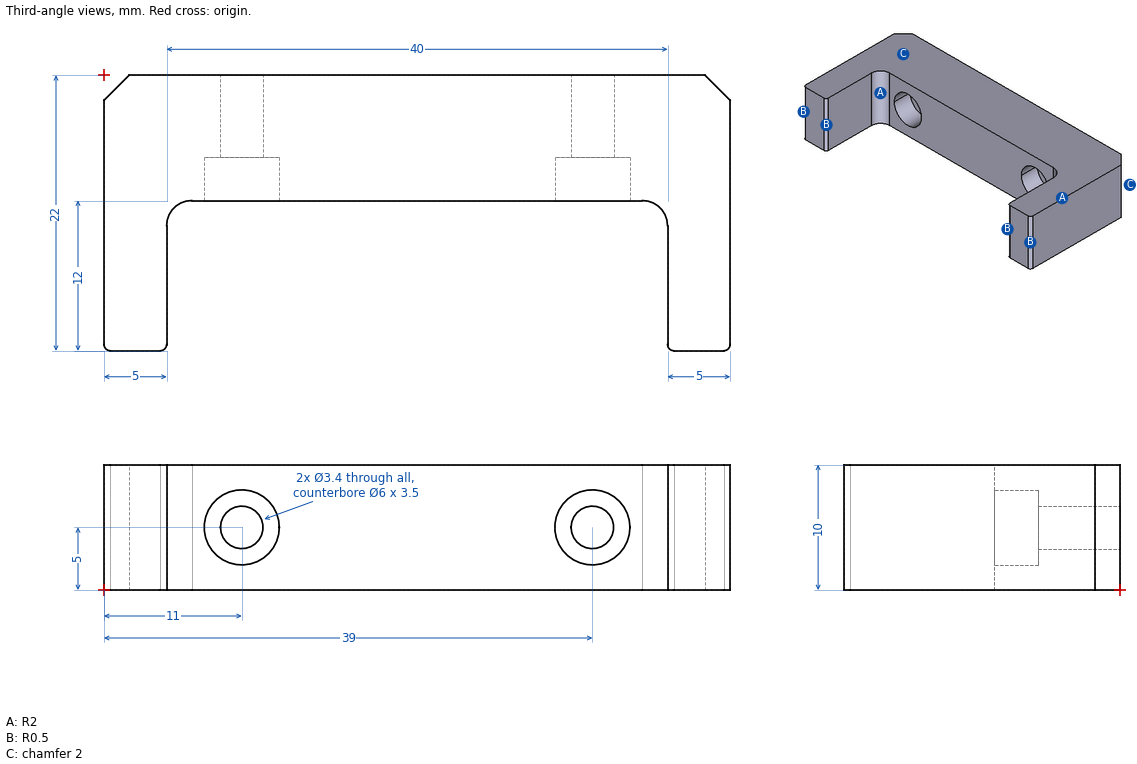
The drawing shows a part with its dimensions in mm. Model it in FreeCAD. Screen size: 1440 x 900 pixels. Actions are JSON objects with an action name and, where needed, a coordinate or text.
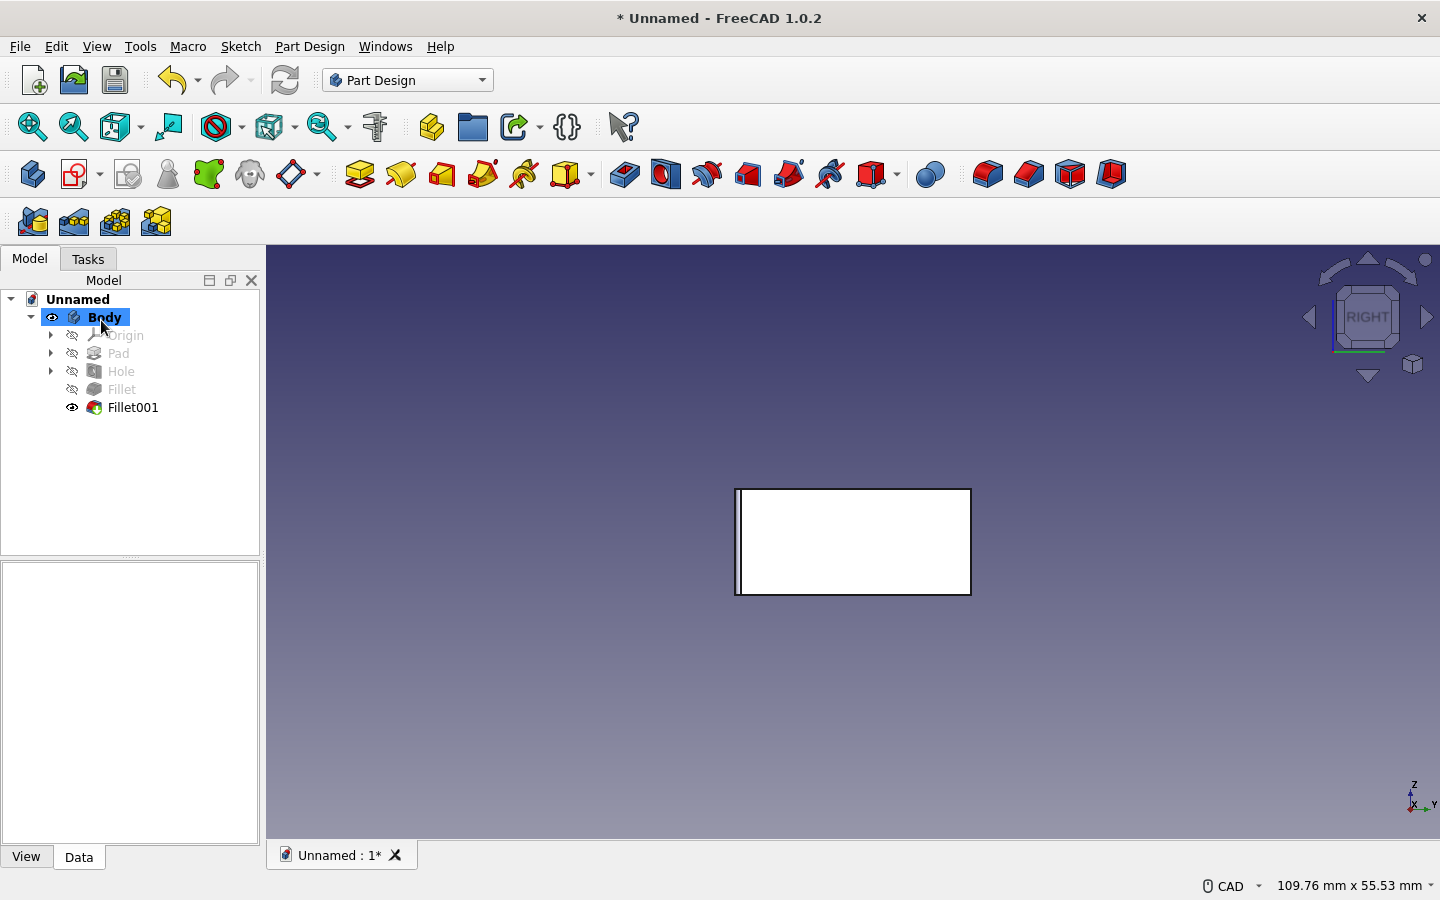
{"action": "left_click", "coordinate": [33, 128]}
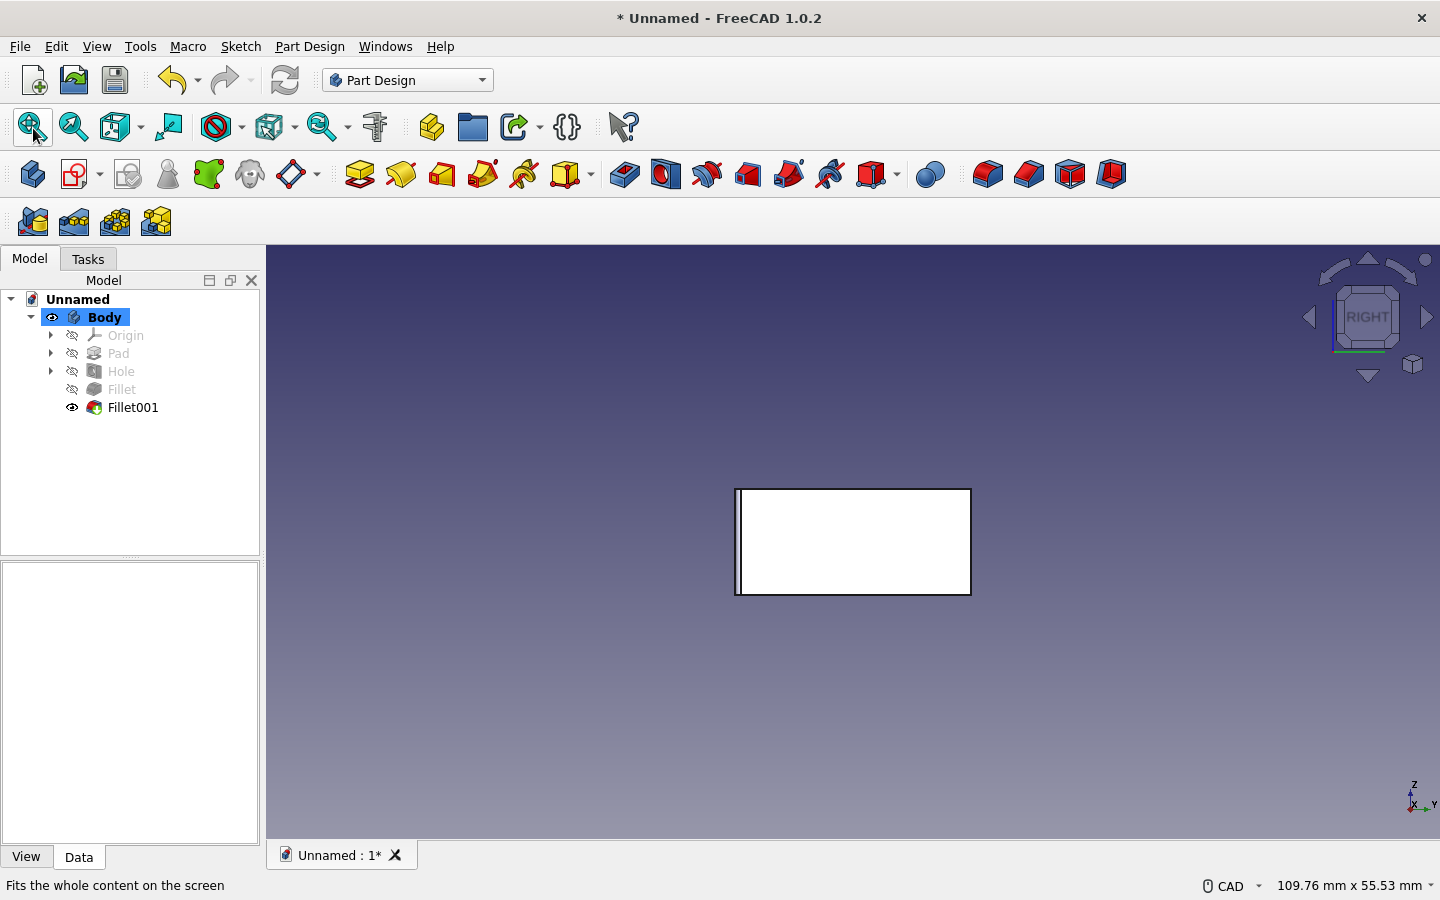
{"action": "left_click", "coordinate": [971, 541]}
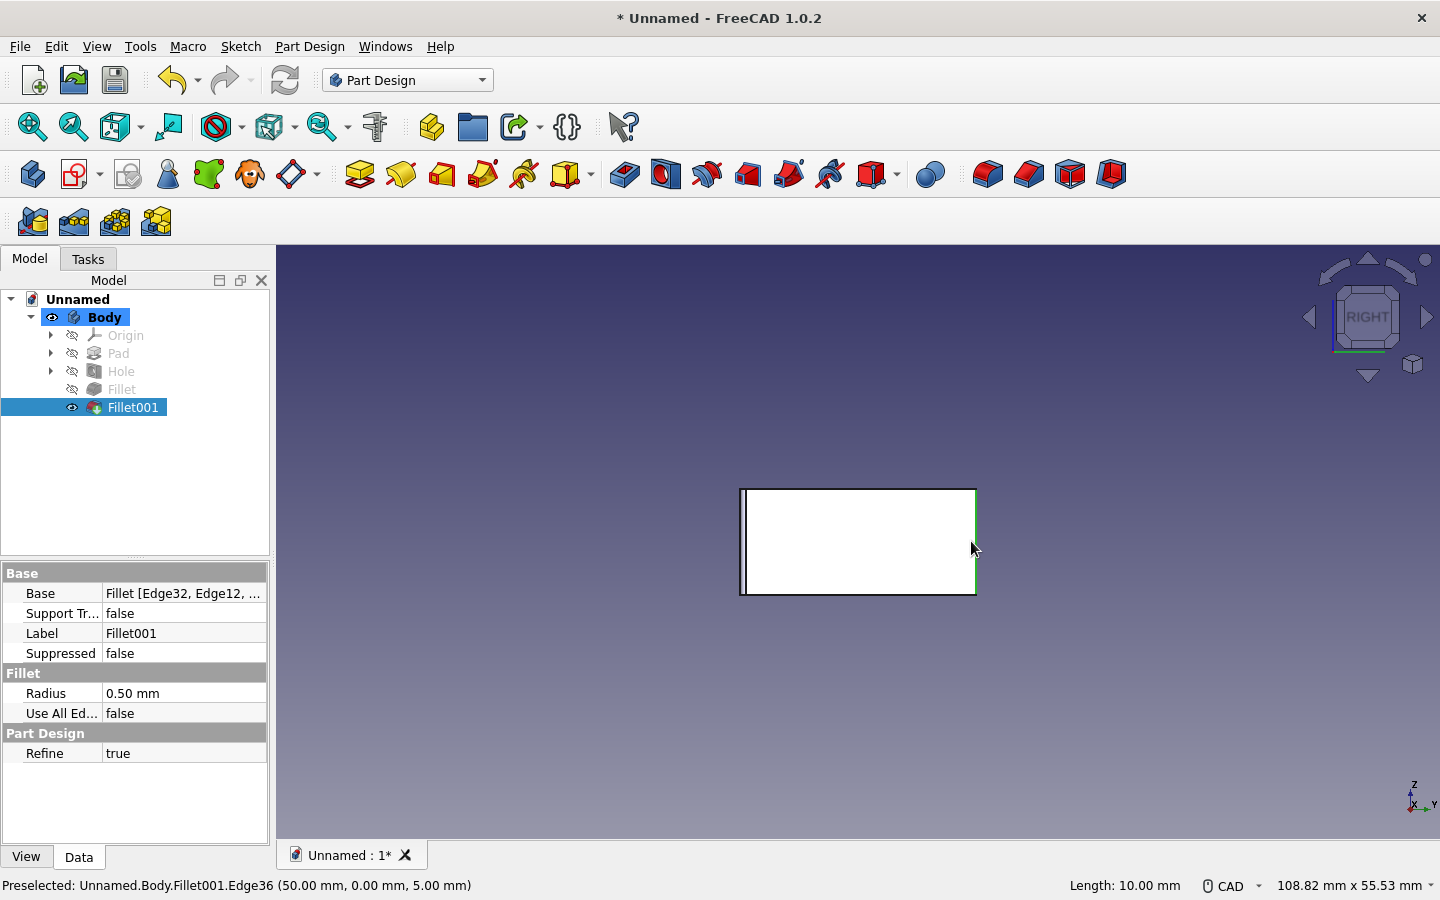
{"action": "key", "text": "5"}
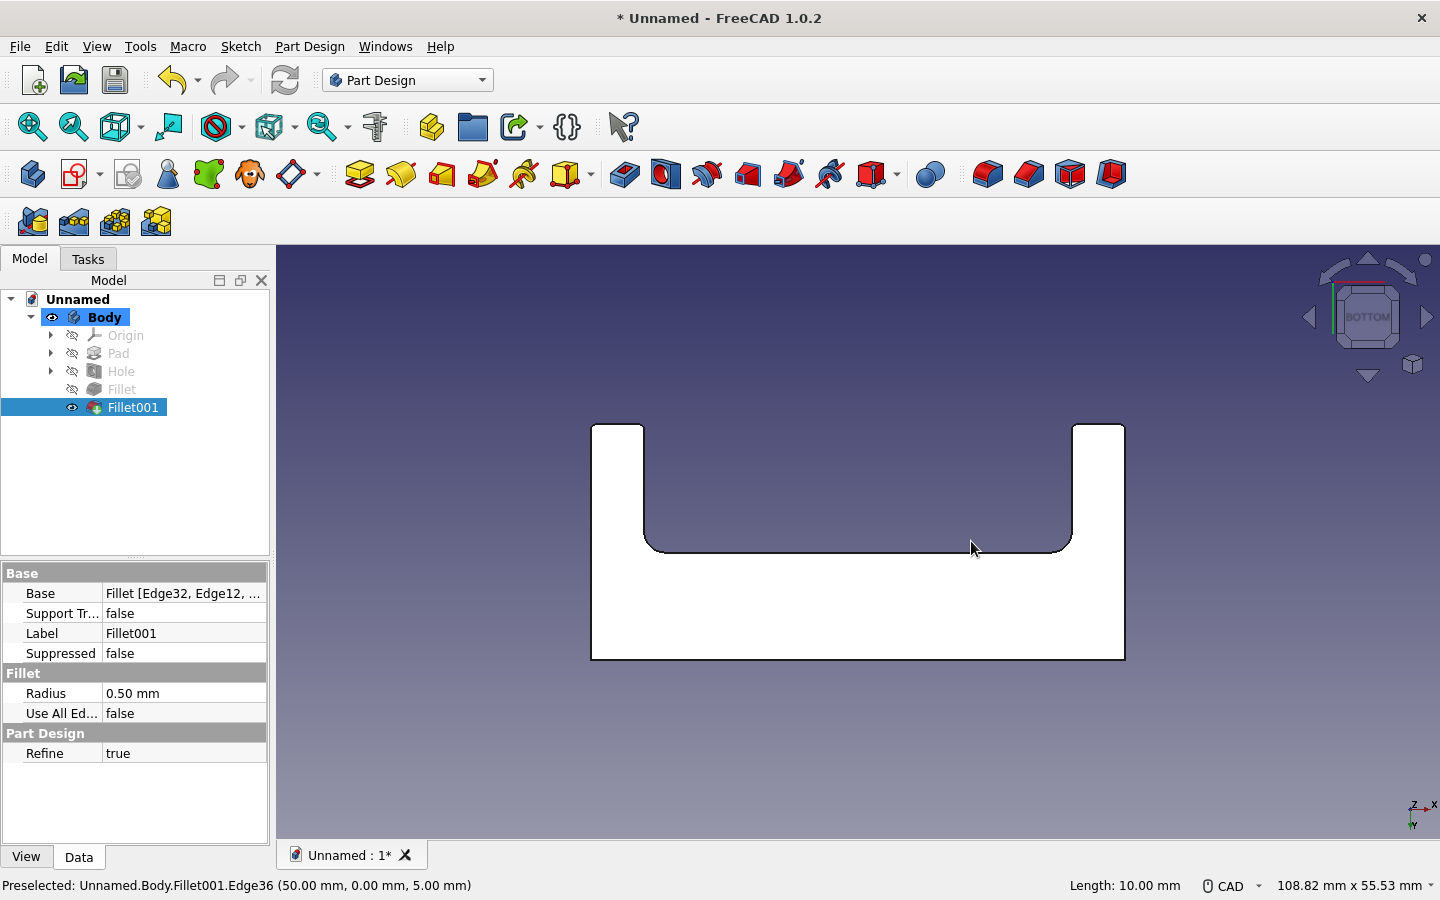
{"action": "key", "text": "4"}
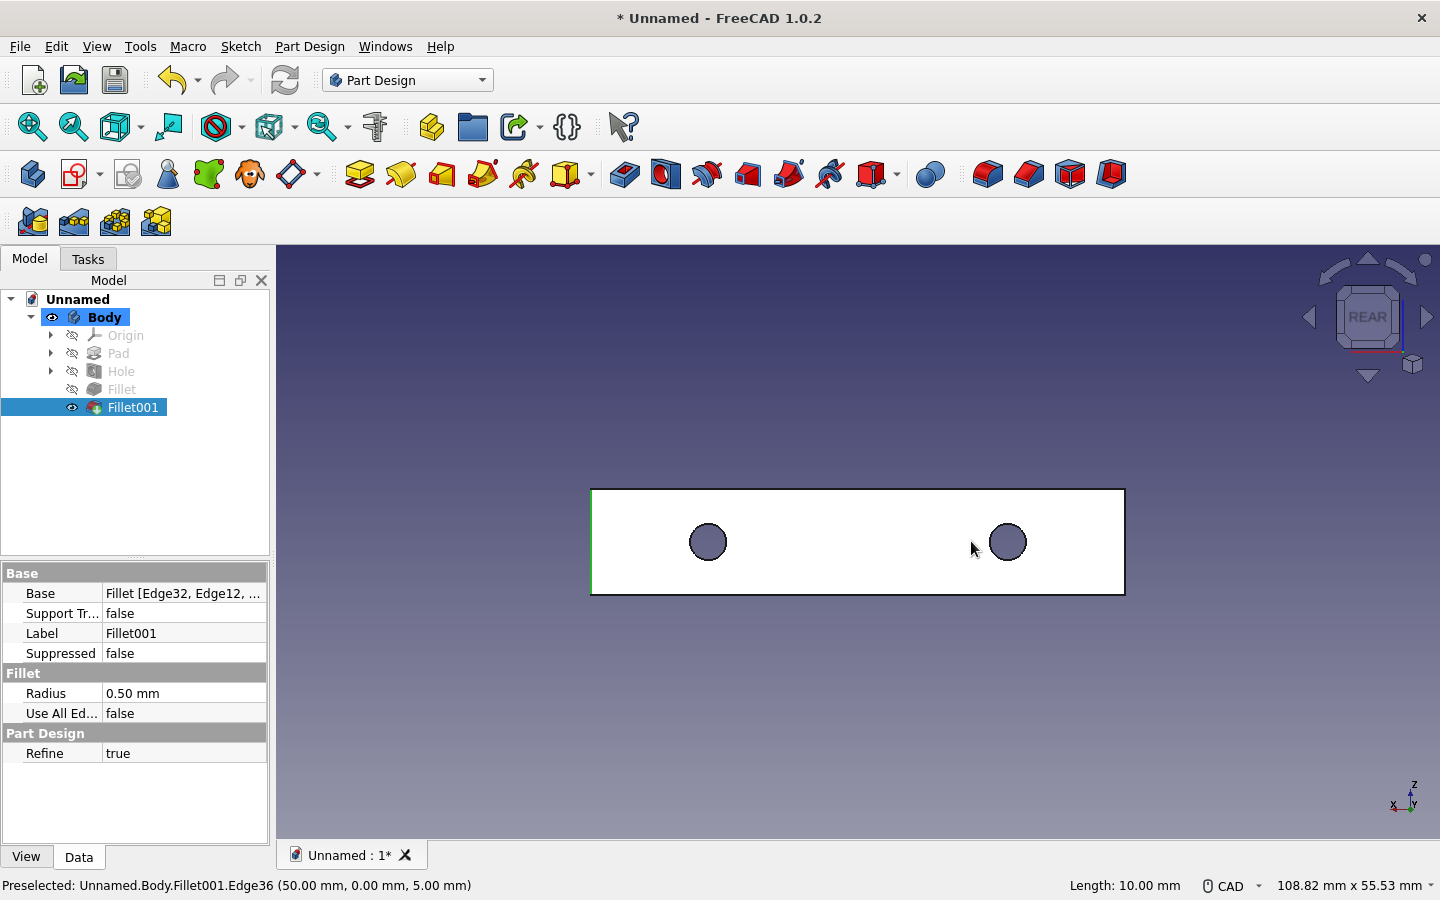
{"action": "left_click", "coordinate": [1125, 541], "text": "ctrl"}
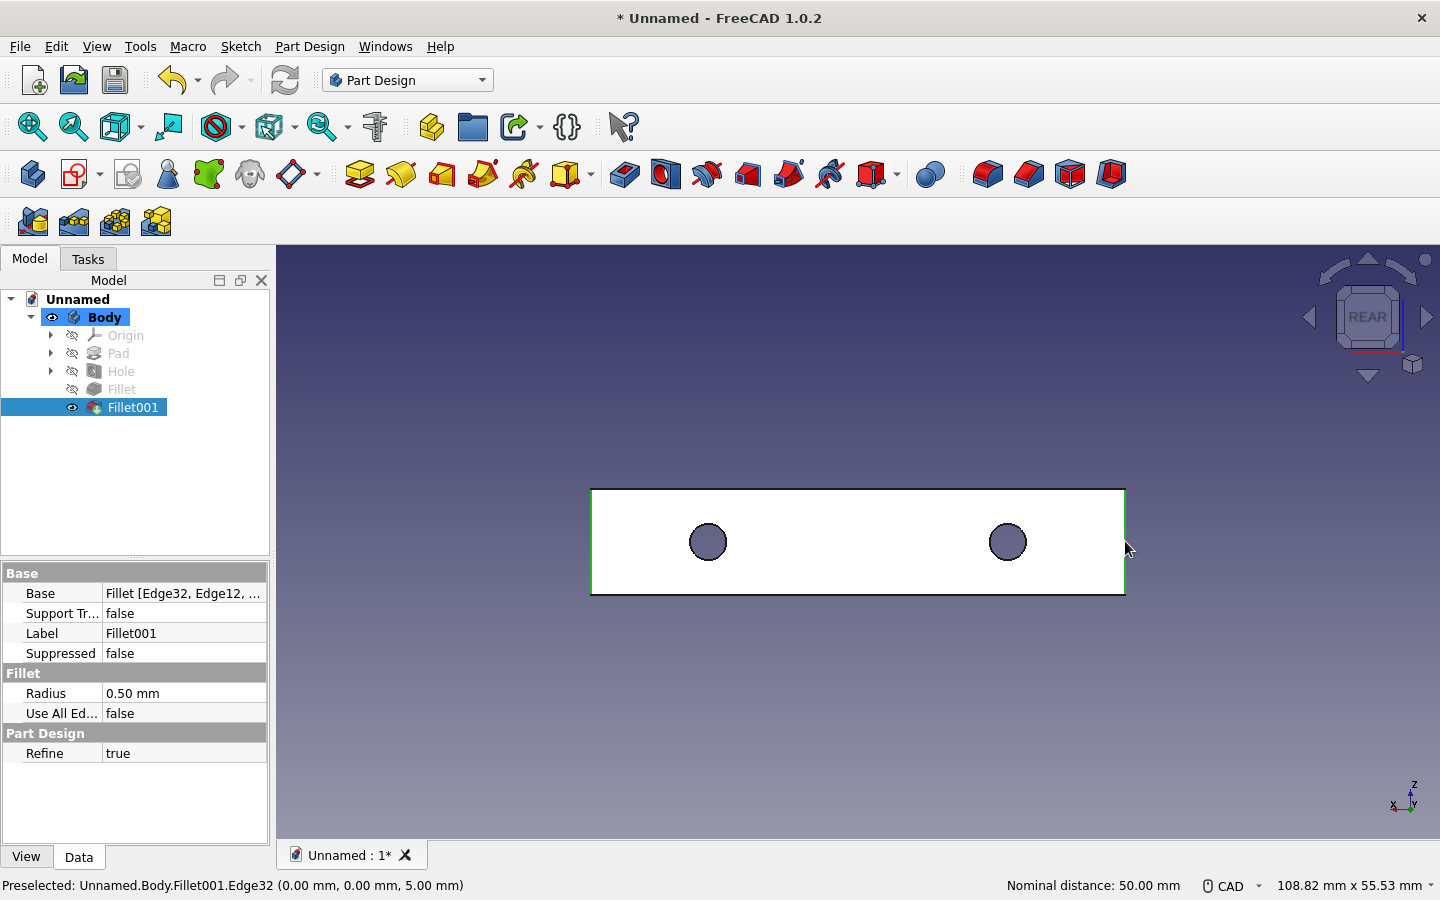
{"action": "left_click", "coordinate": [1029, 174]}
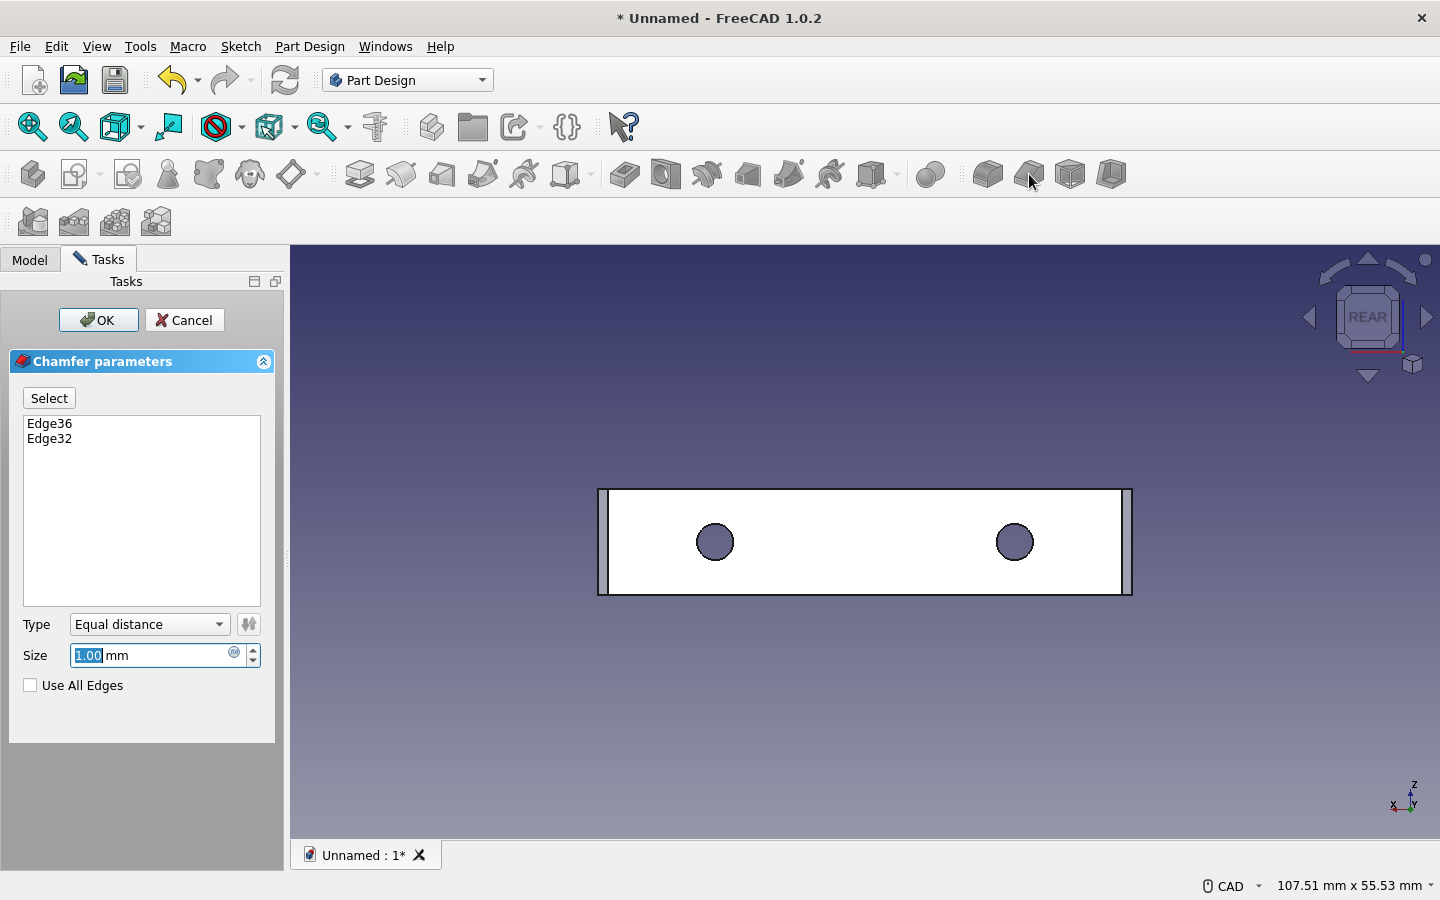
{"action": "type", "text": "2"}
{"action": "key", "text": "Tab"}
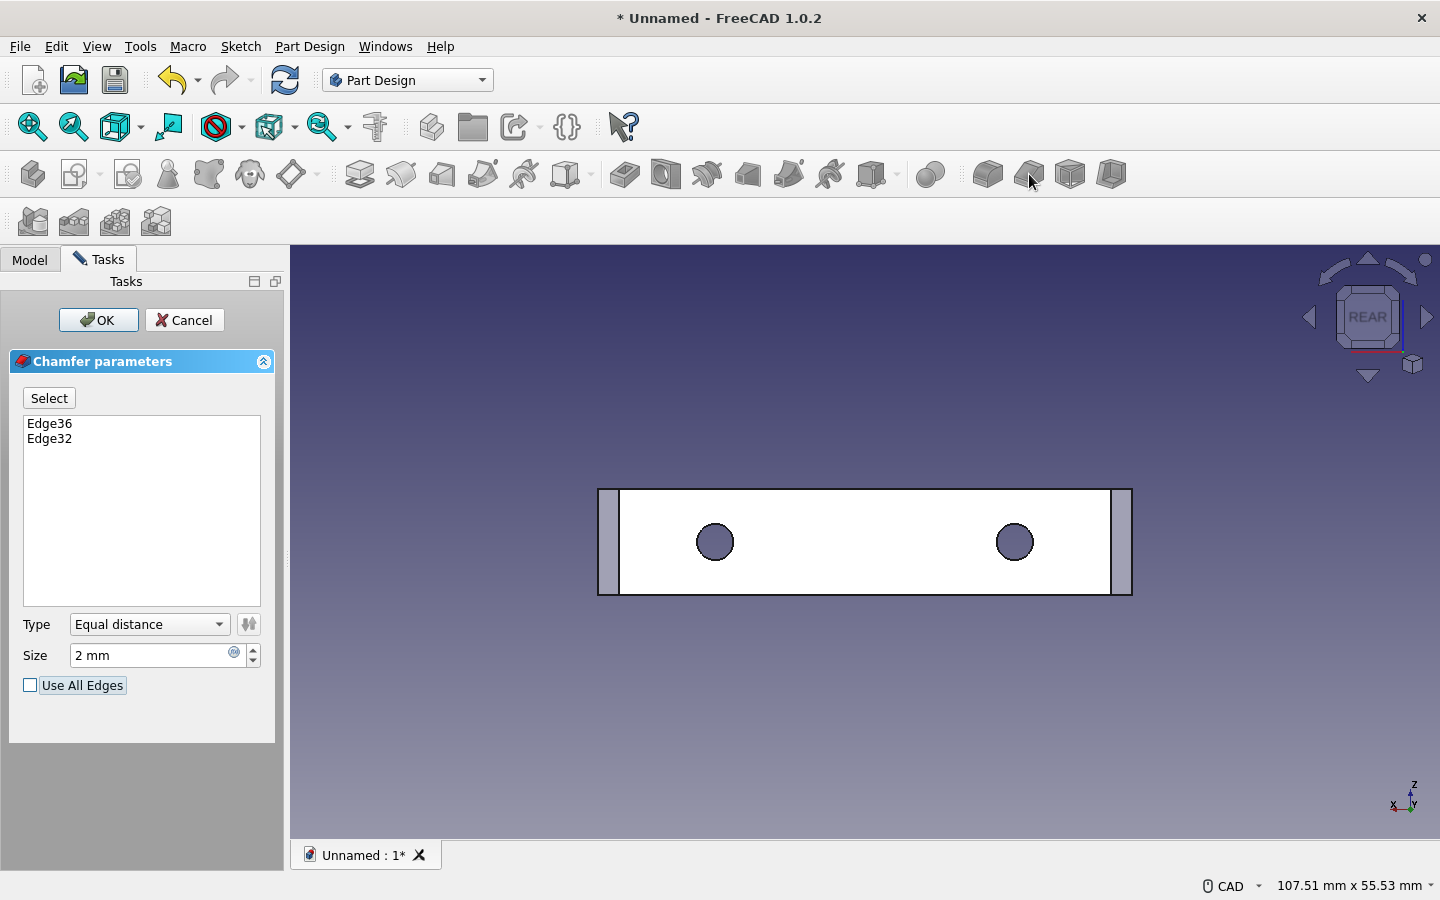
{"action": "left_click", "coordinate": [99, 320]}